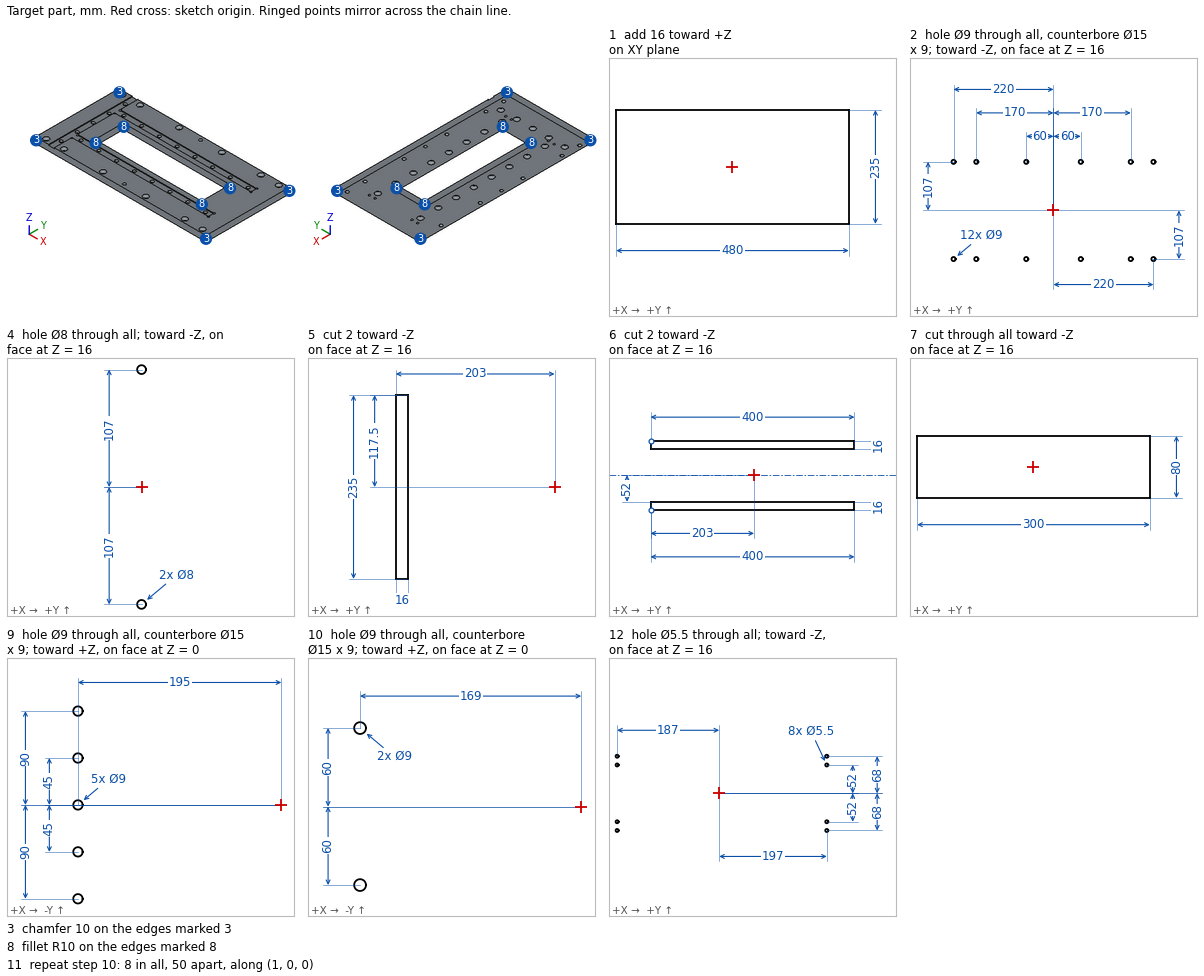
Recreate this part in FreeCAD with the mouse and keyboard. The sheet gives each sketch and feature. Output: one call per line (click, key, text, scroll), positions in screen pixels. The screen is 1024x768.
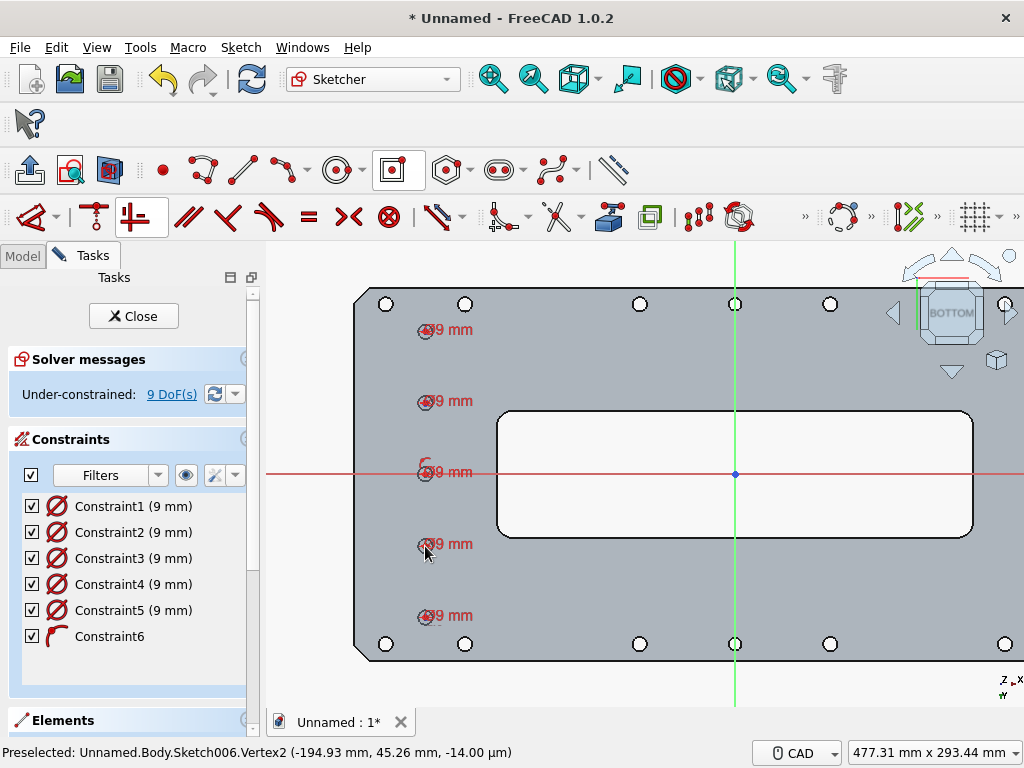
click(162, 218)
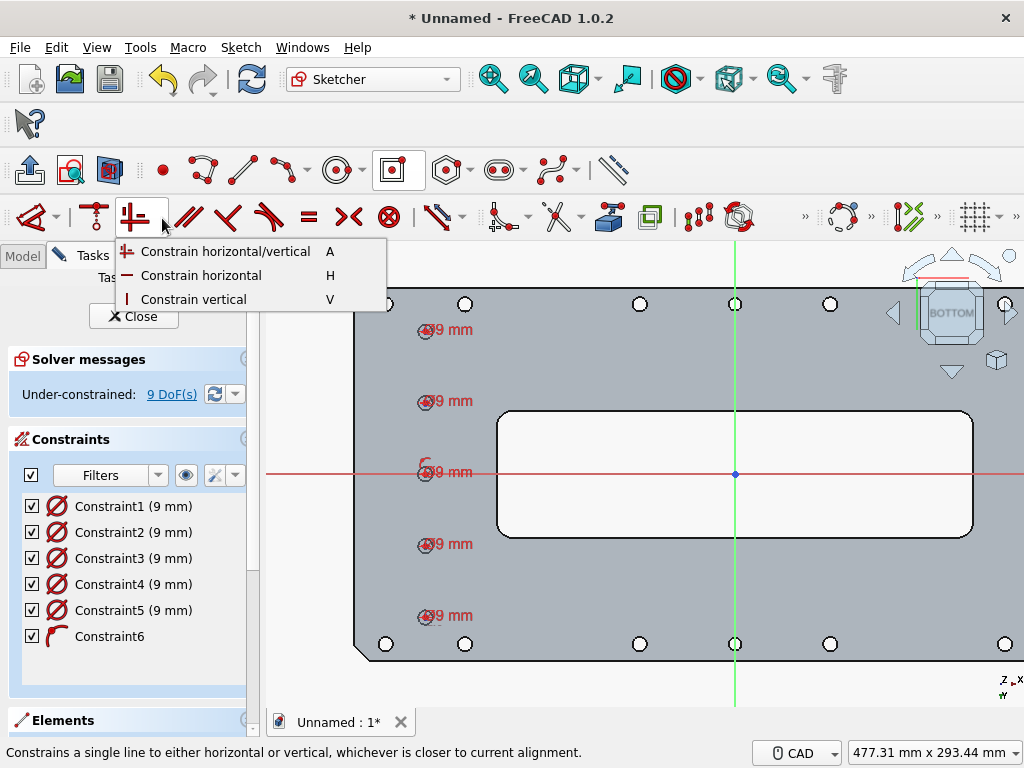
click(251, 299)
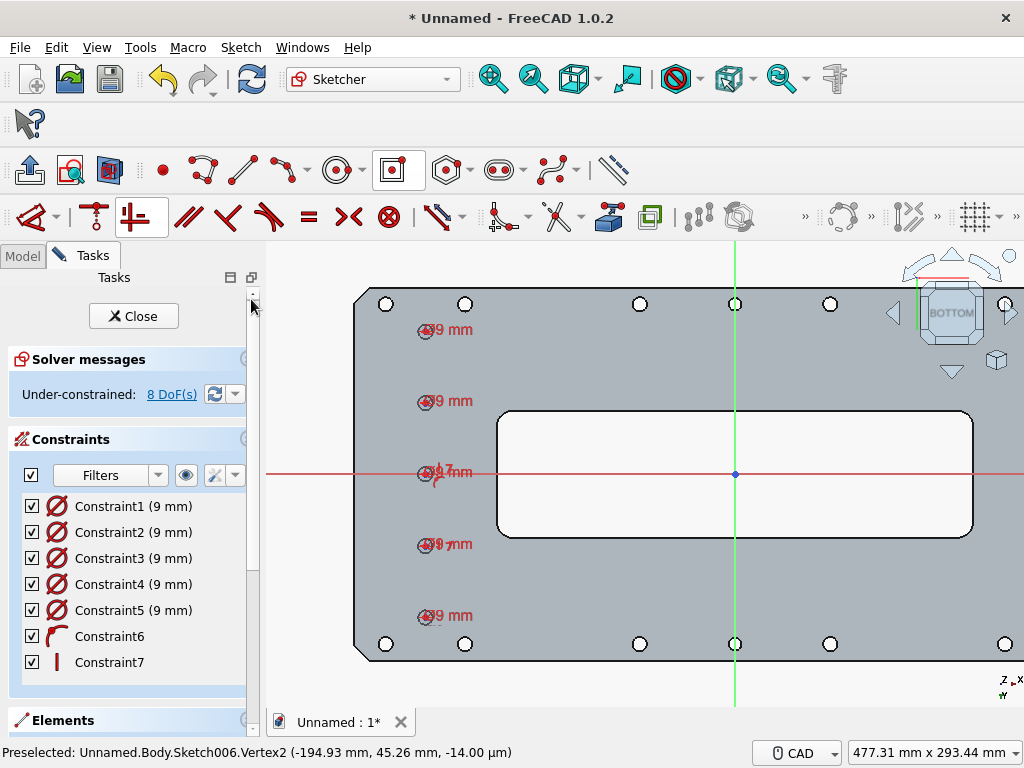
click(425, 546)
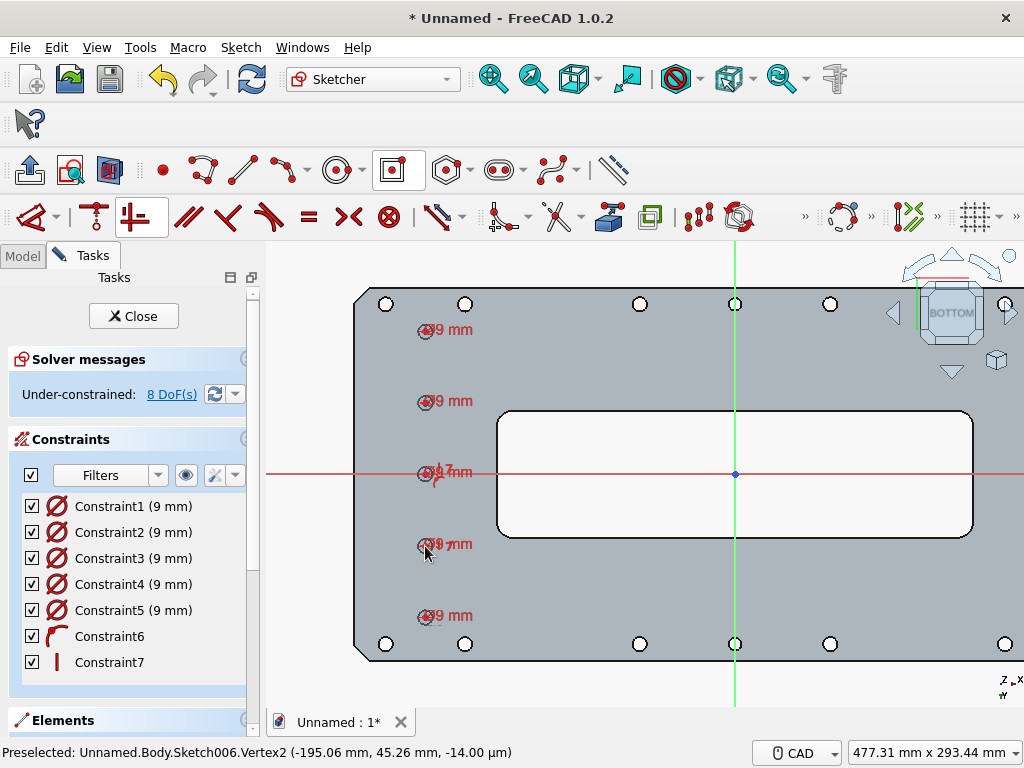
click(425, 618)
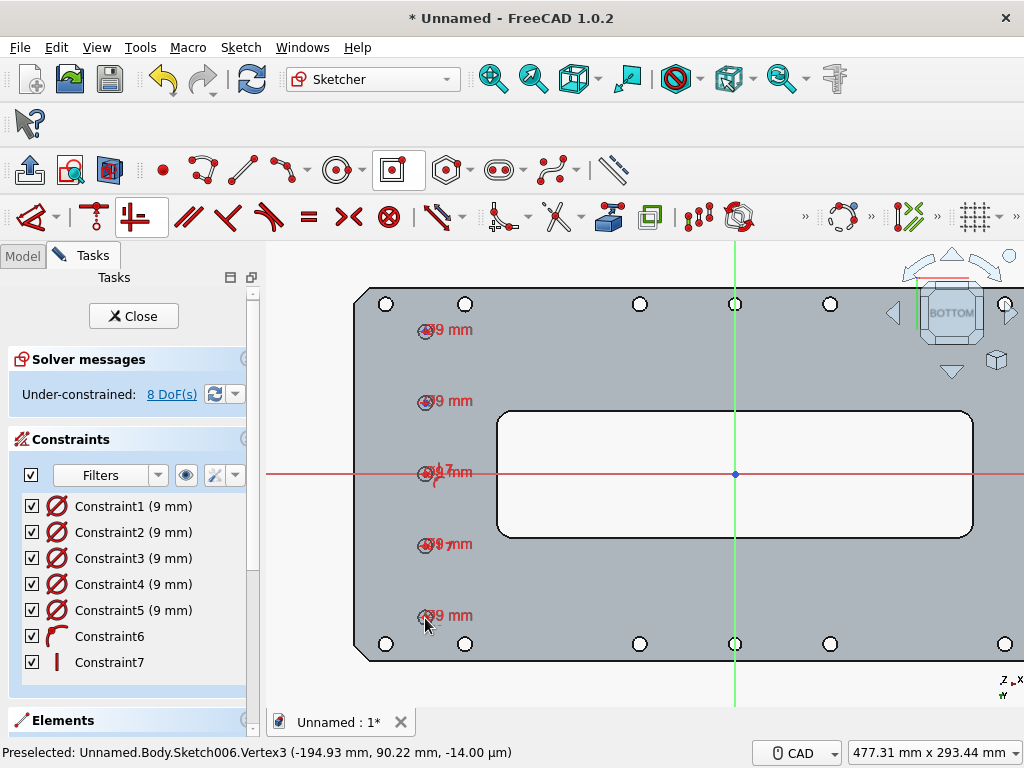
click(162, 218)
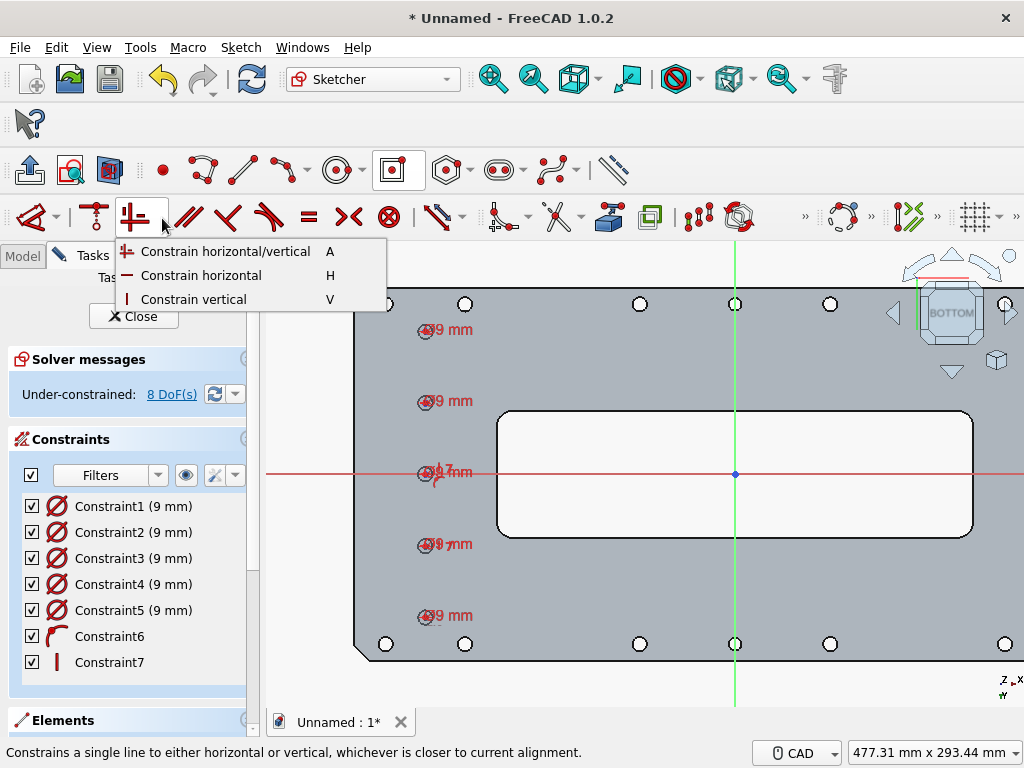
click(251, 299)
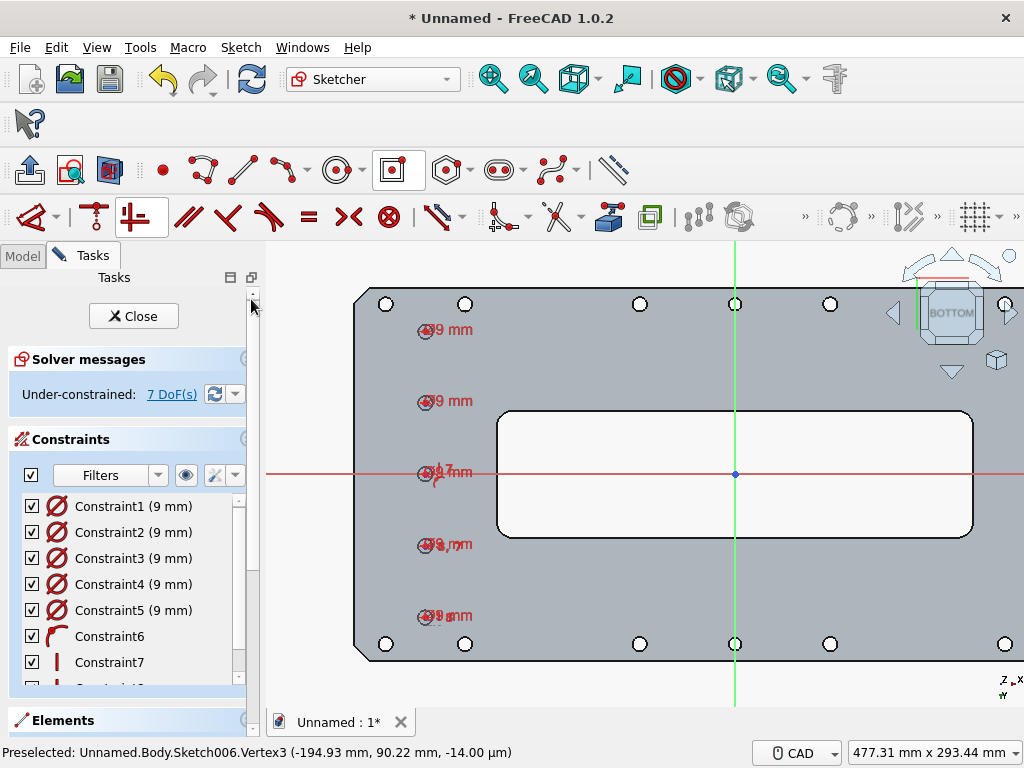
click(425, 474)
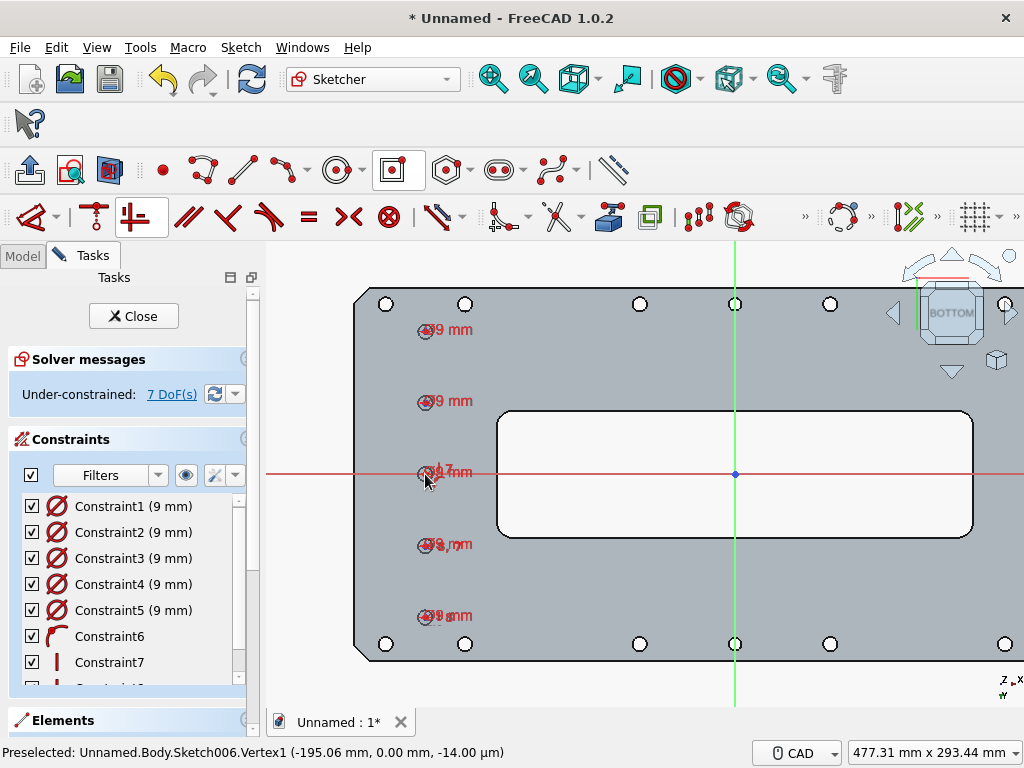
click(425, 332)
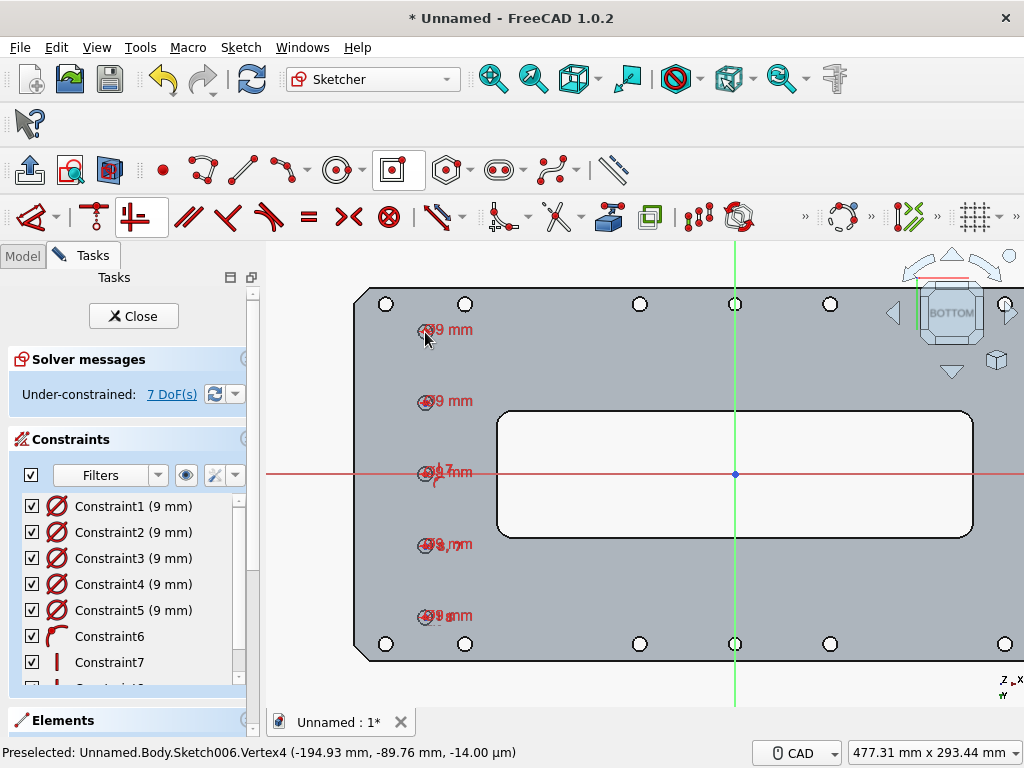
click(162, 218)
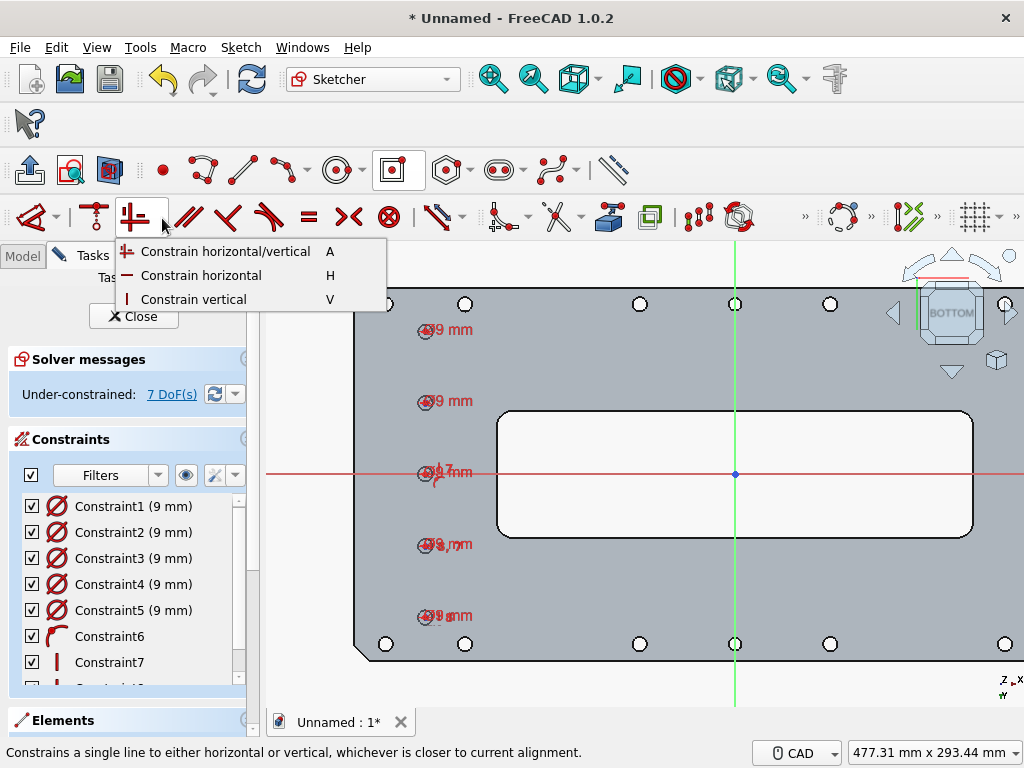
click(251, 299)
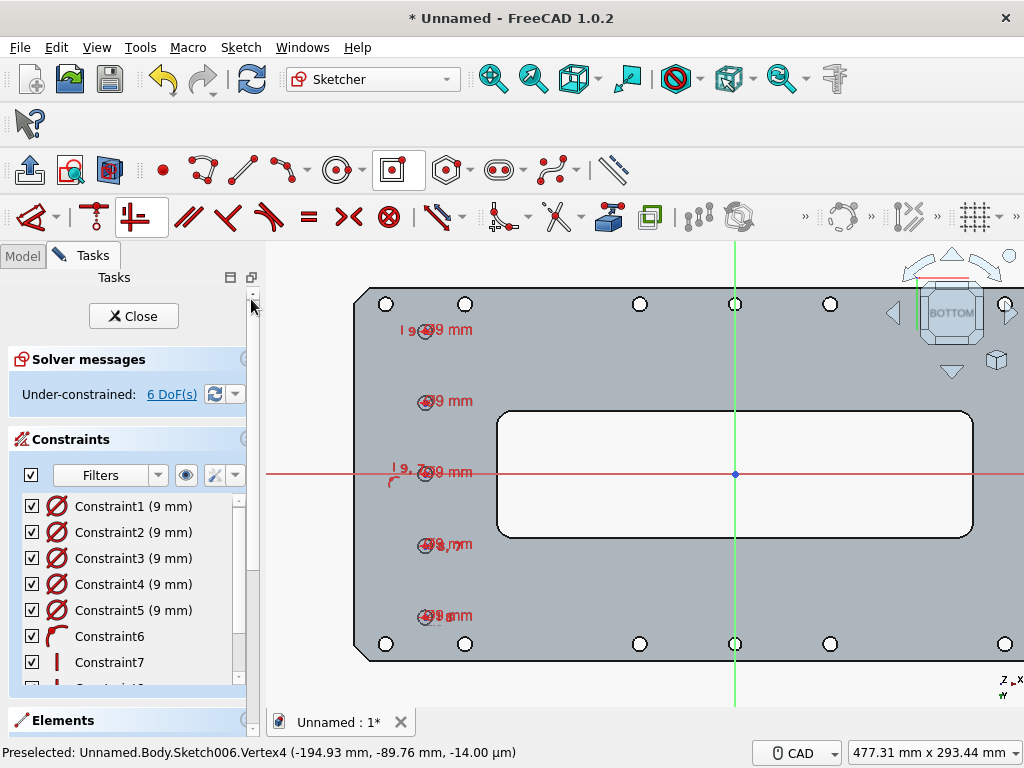
click(425, 474)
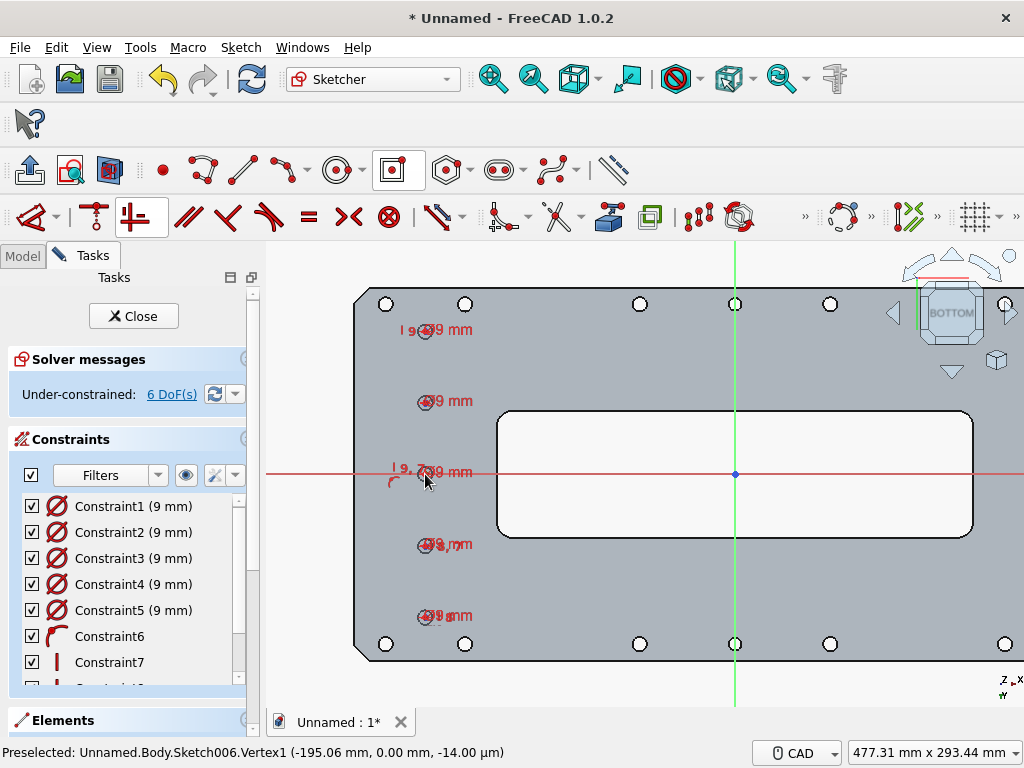
click(425, 403)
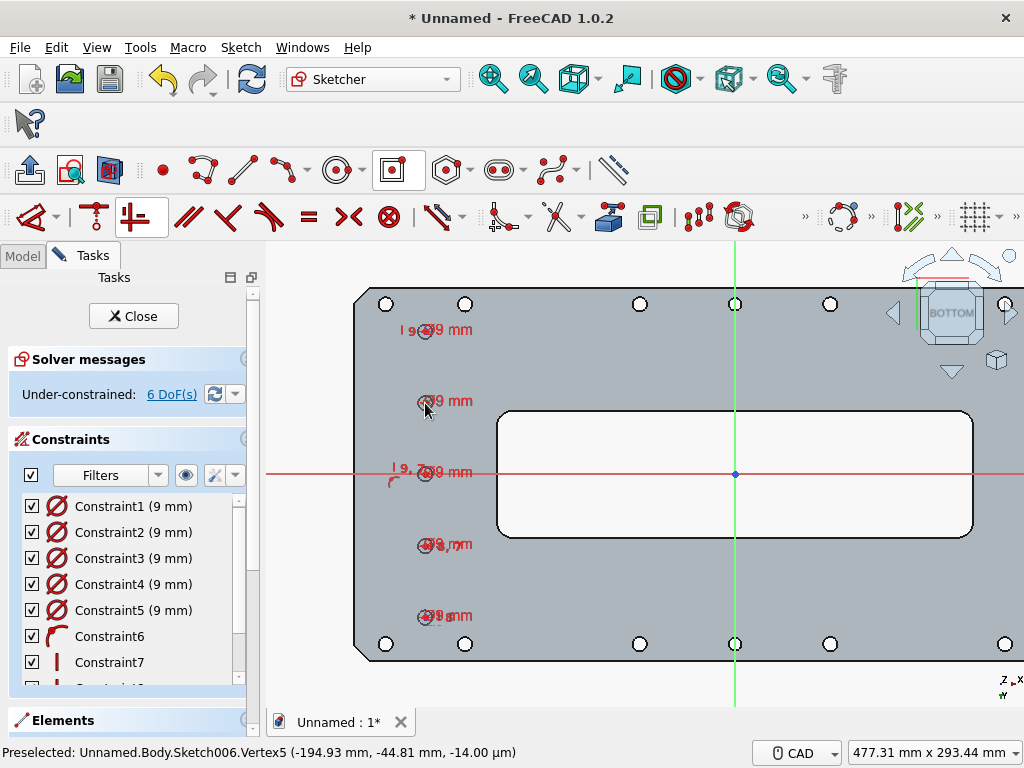
key(v)